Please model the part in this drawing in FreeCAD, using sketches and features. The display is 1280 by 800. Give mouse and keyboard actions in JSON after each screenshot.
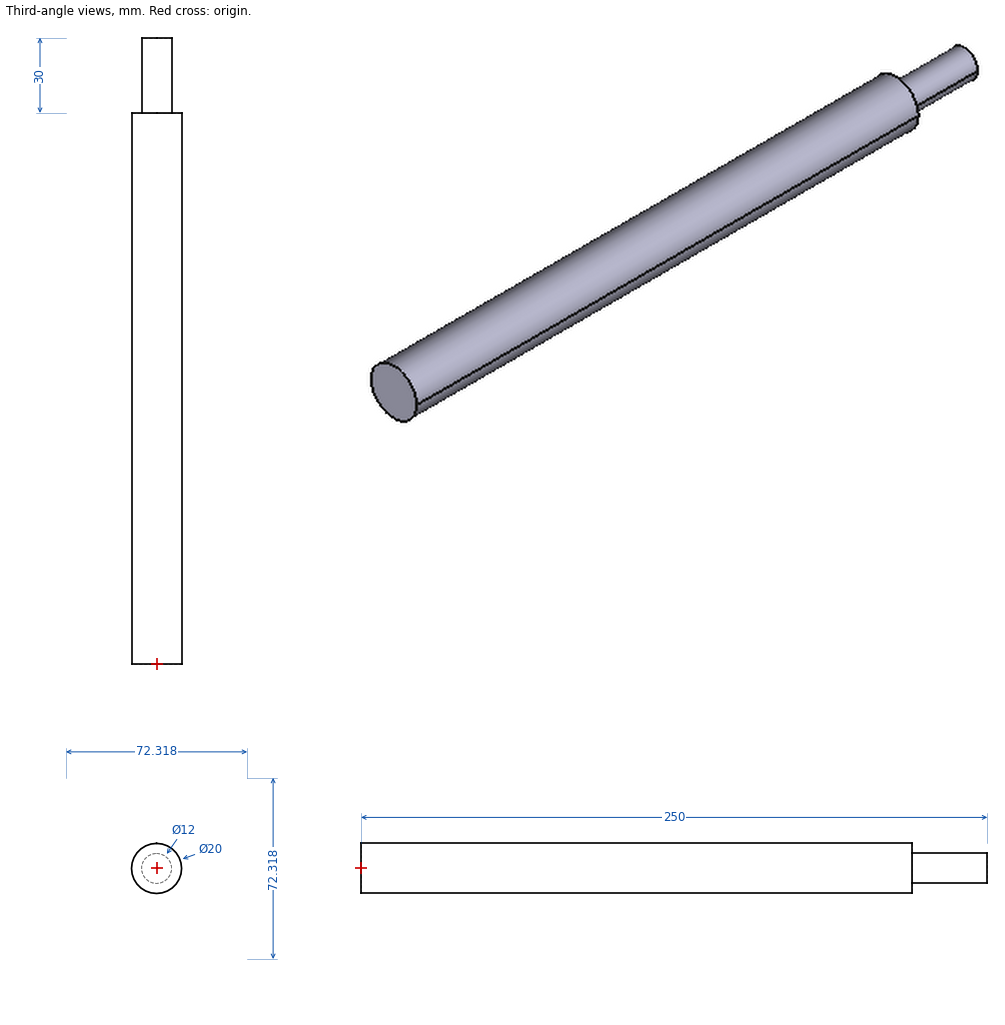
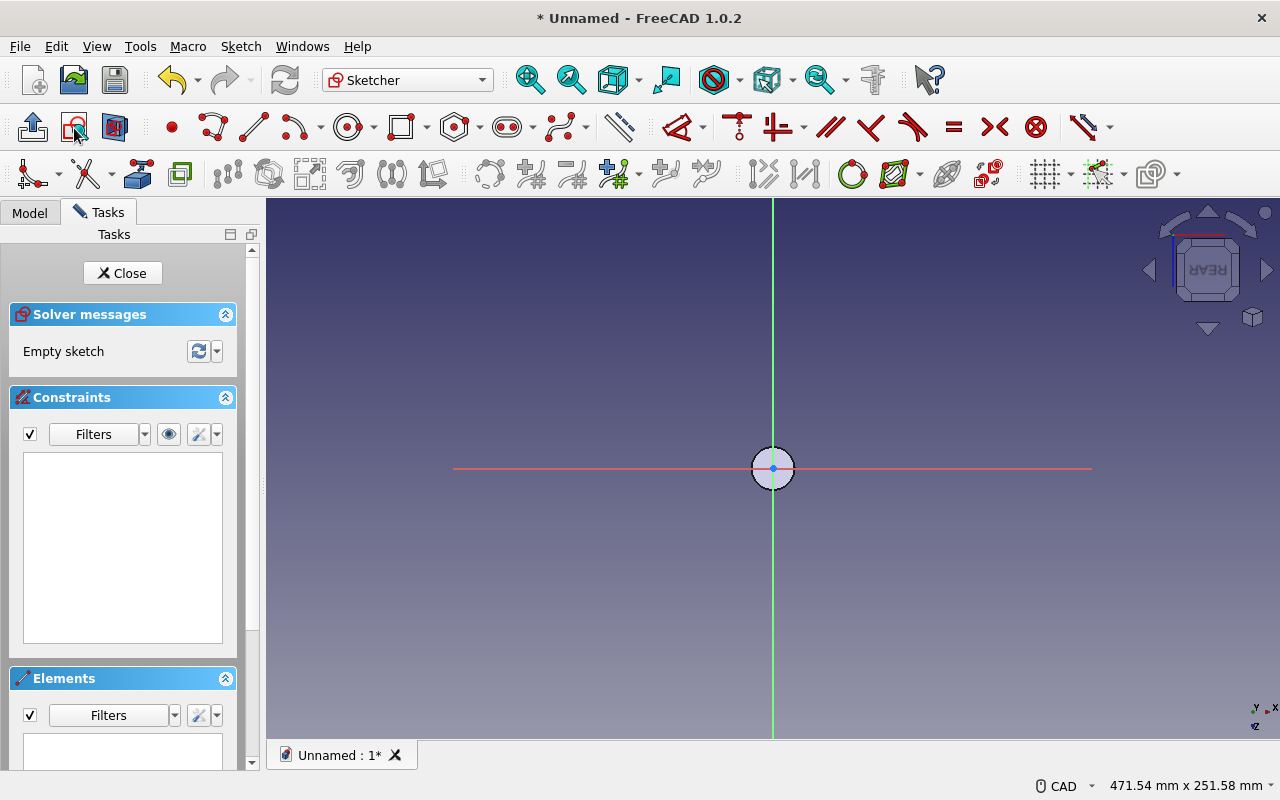
{"action": "scroll", "coordinate": [829, 468], "scroll_direction": "up", "scroll_amount": 4}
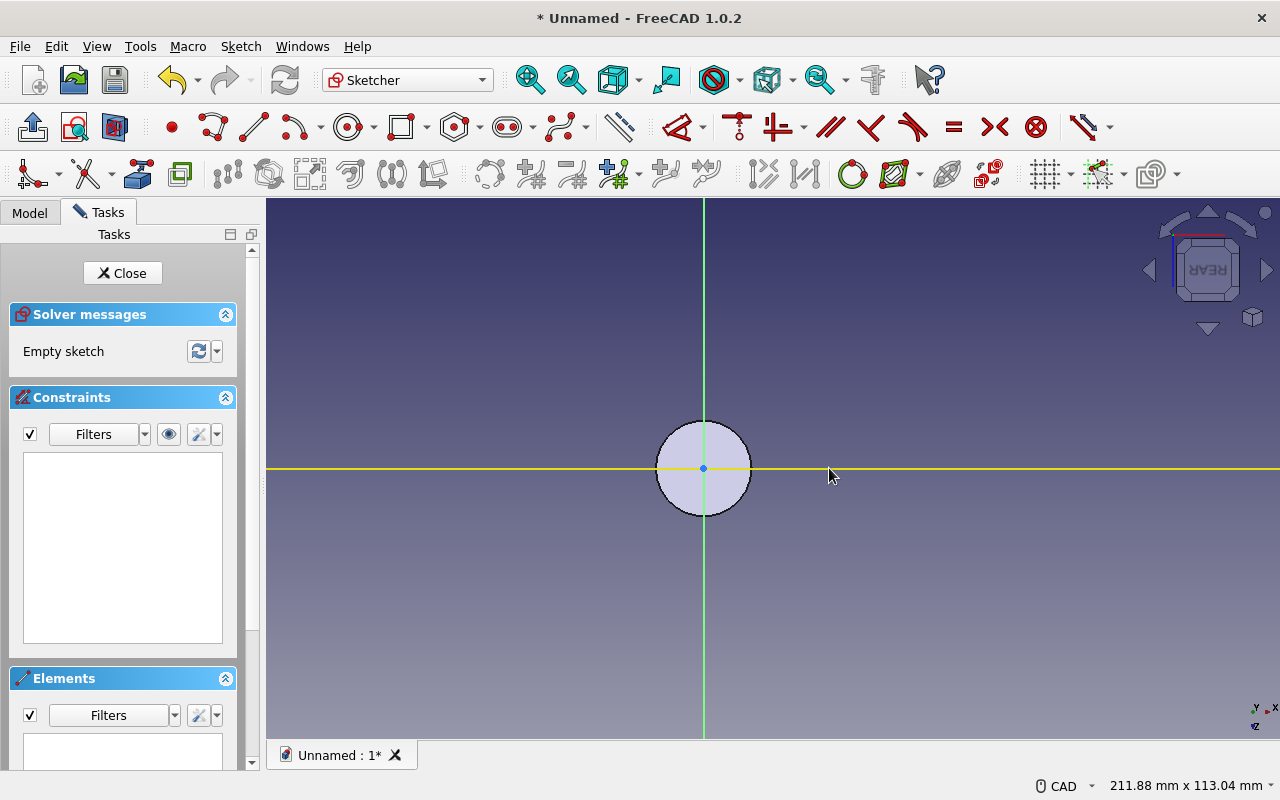
{"action": "key", "text": "g v"}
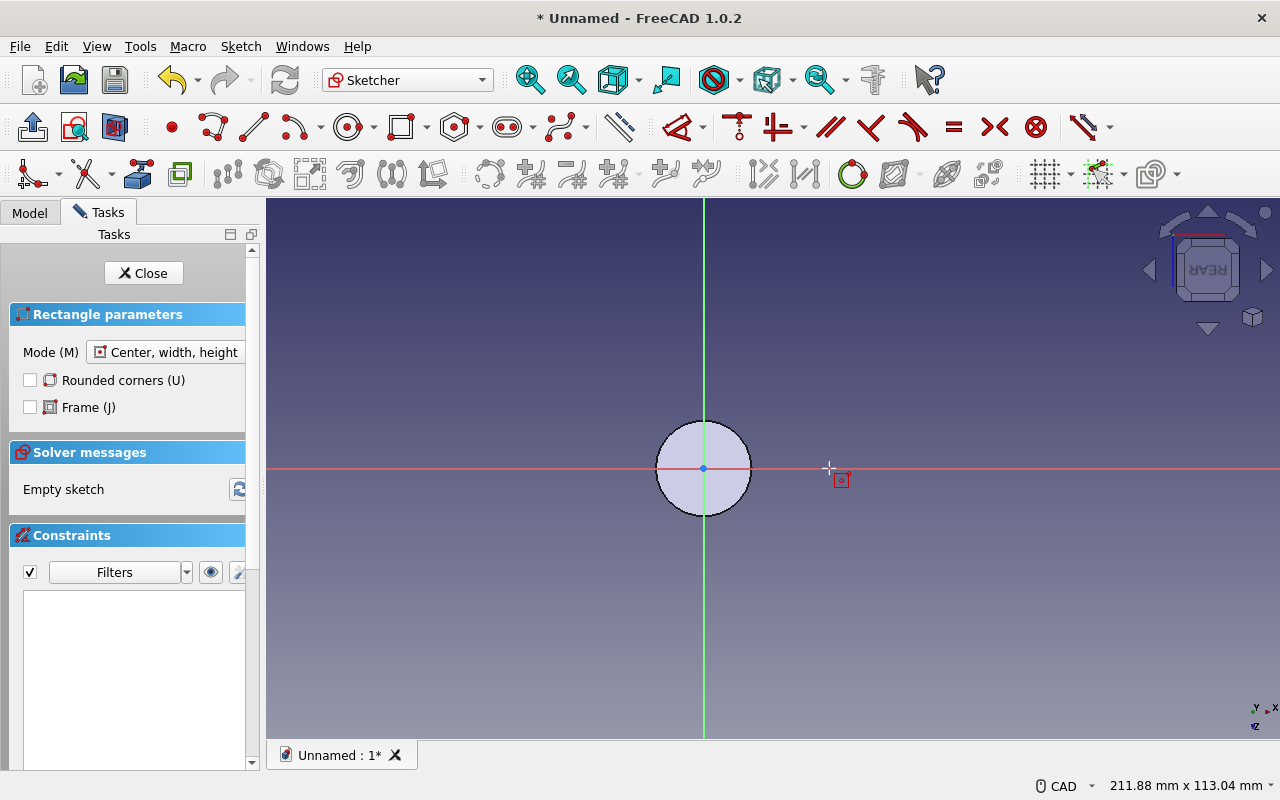
{"action": "left_click", "coordinate": [704, 468]}
{"action": "left_click", "coordinate": [877, 295]}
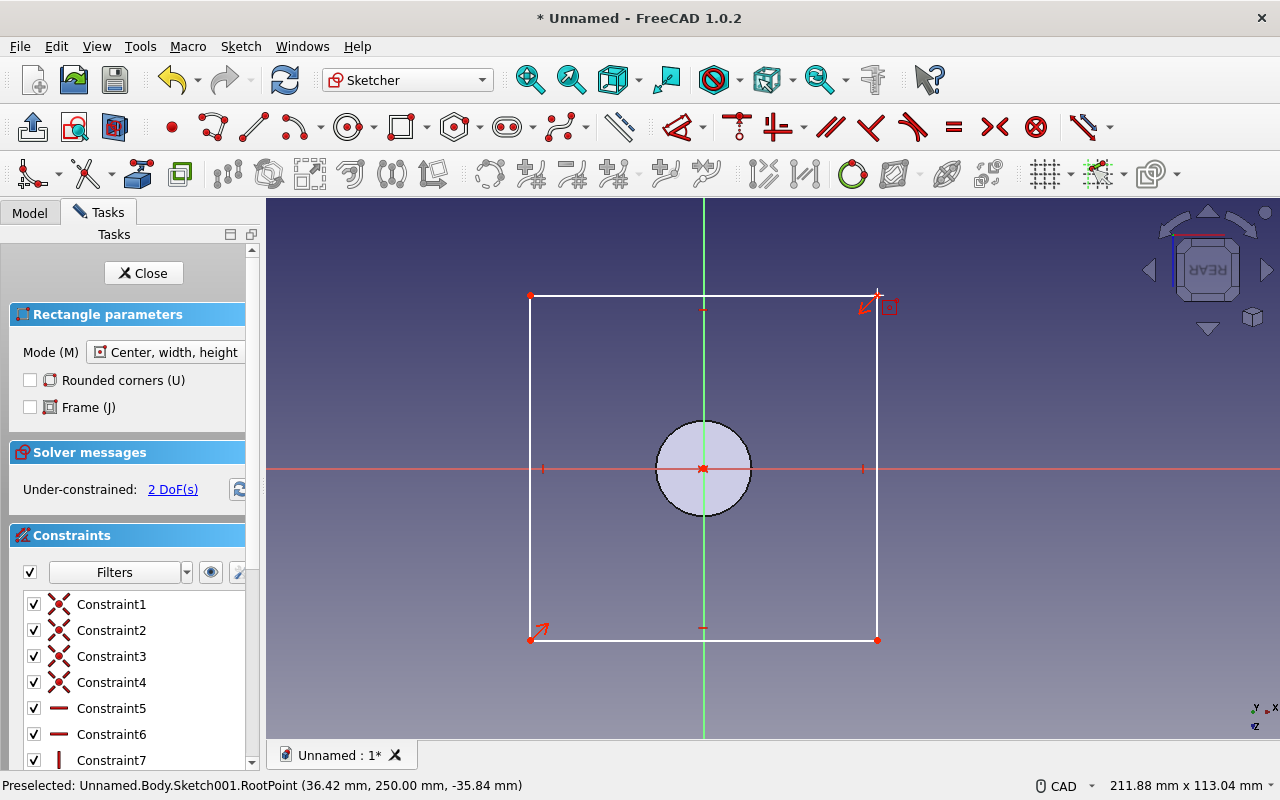
{"action": "left_click", "coordinate": [348, 128]}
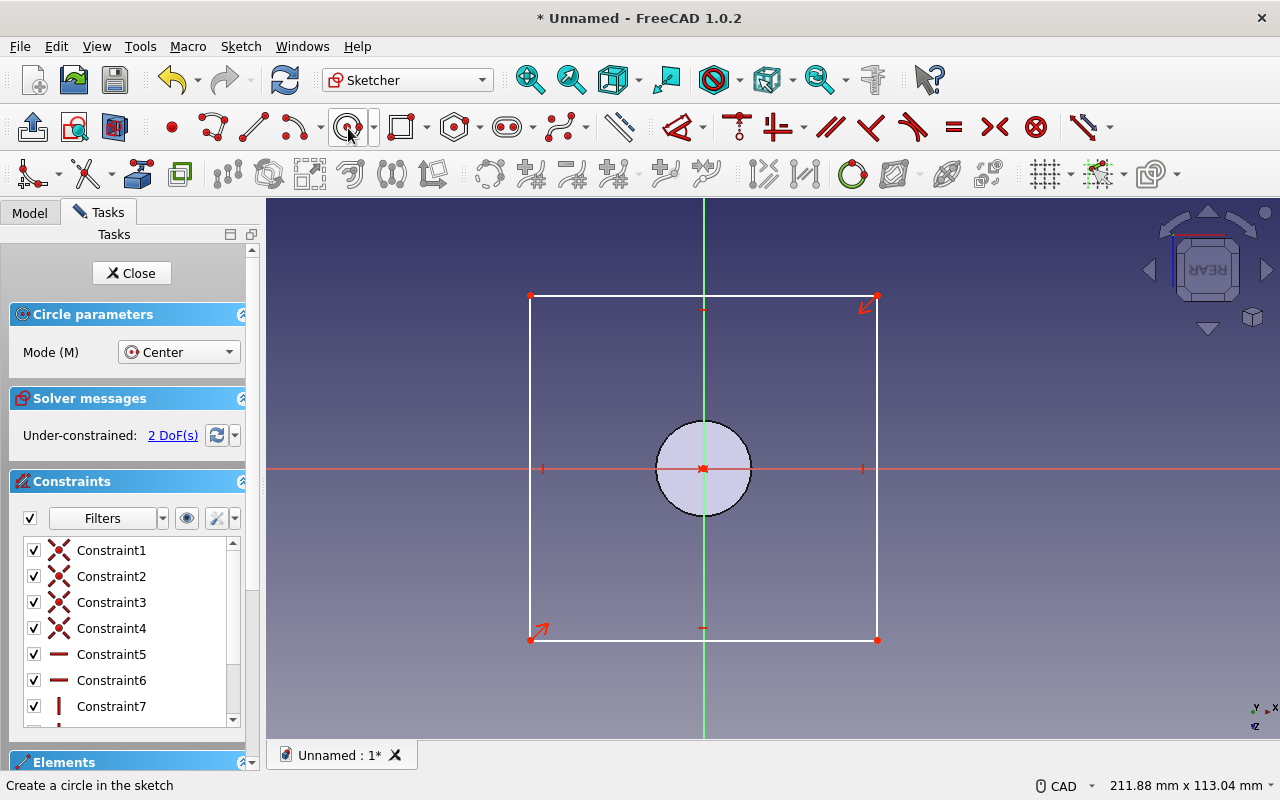
{"action": "left_click", "coordinate": [704, 468]}
{"action": "left_click", "coordinate": [724, 448]}
{"action": "key", "text": "Escape"}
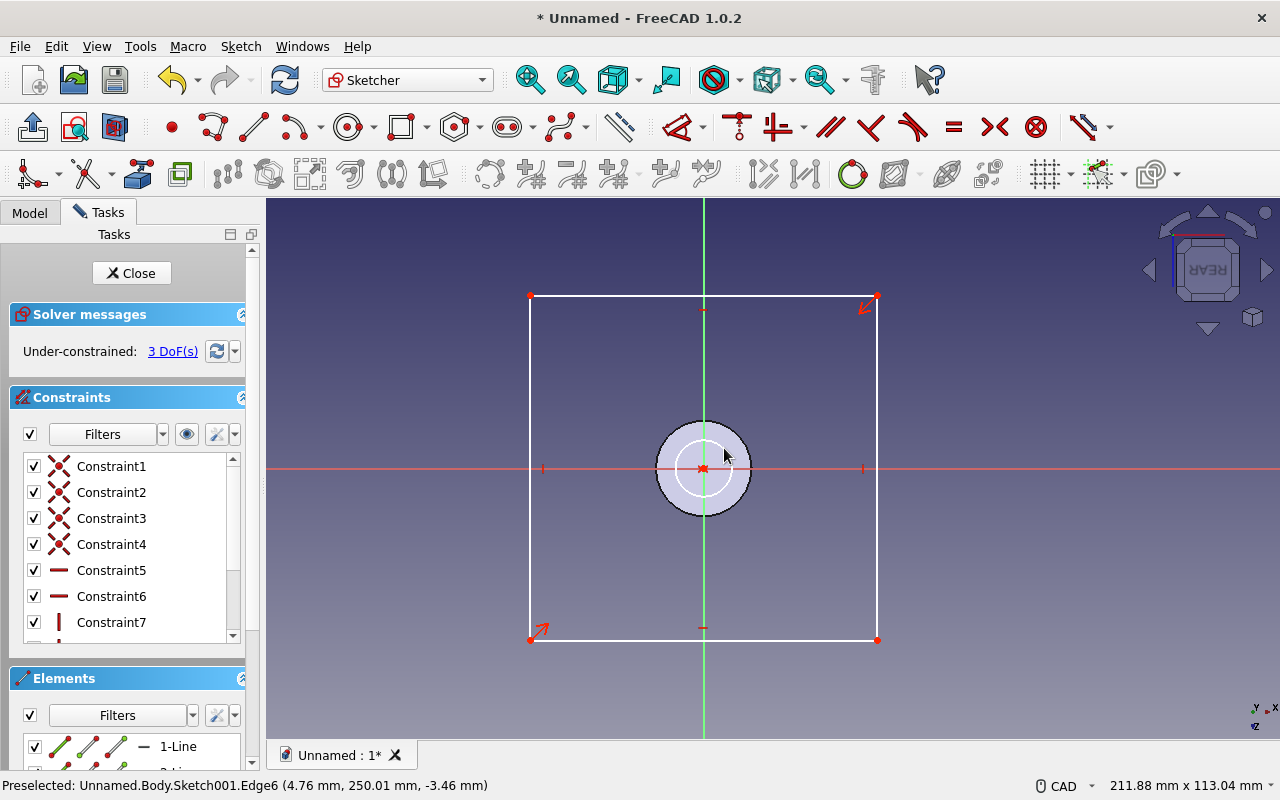
{"action": "left_click", "coordinate": [676, 128]}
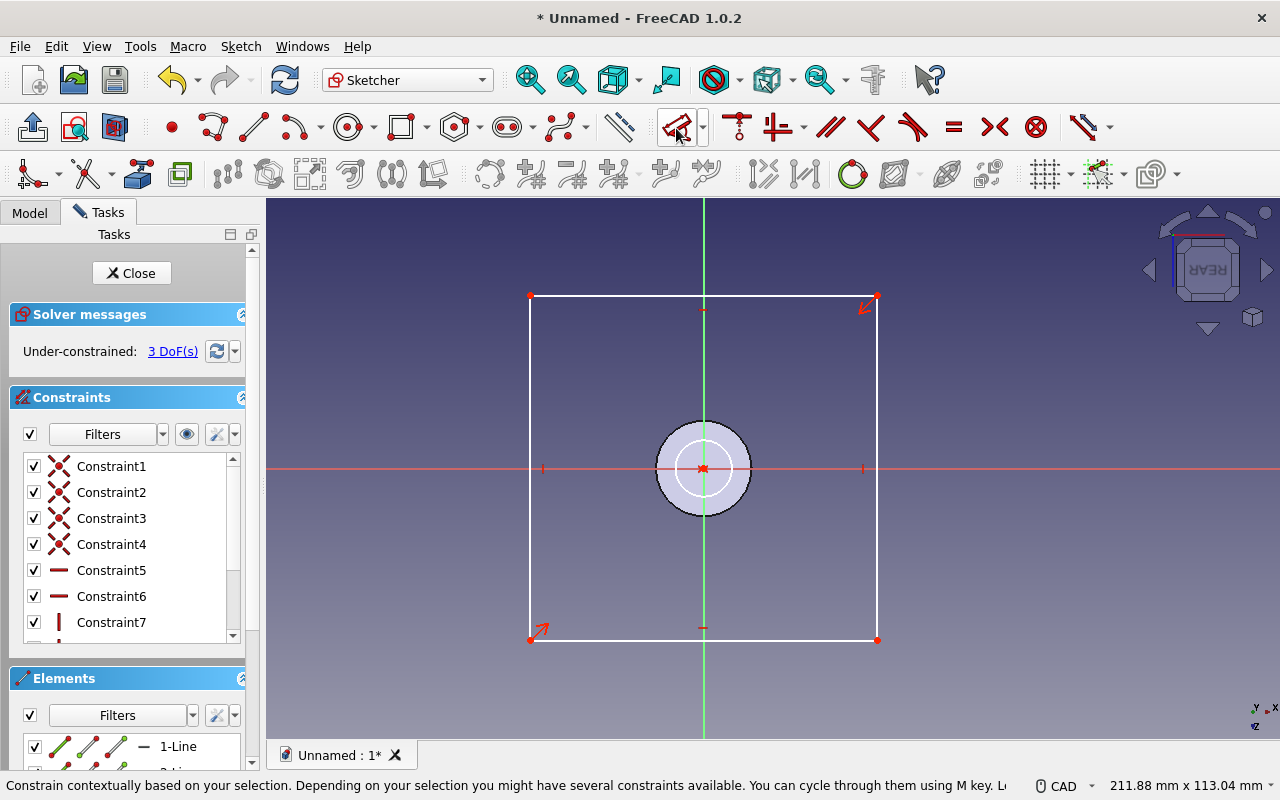
{"action": "left_click", "coordinate": [724, 449]}
{"action": "left_click", "coordinate": [747, 427]}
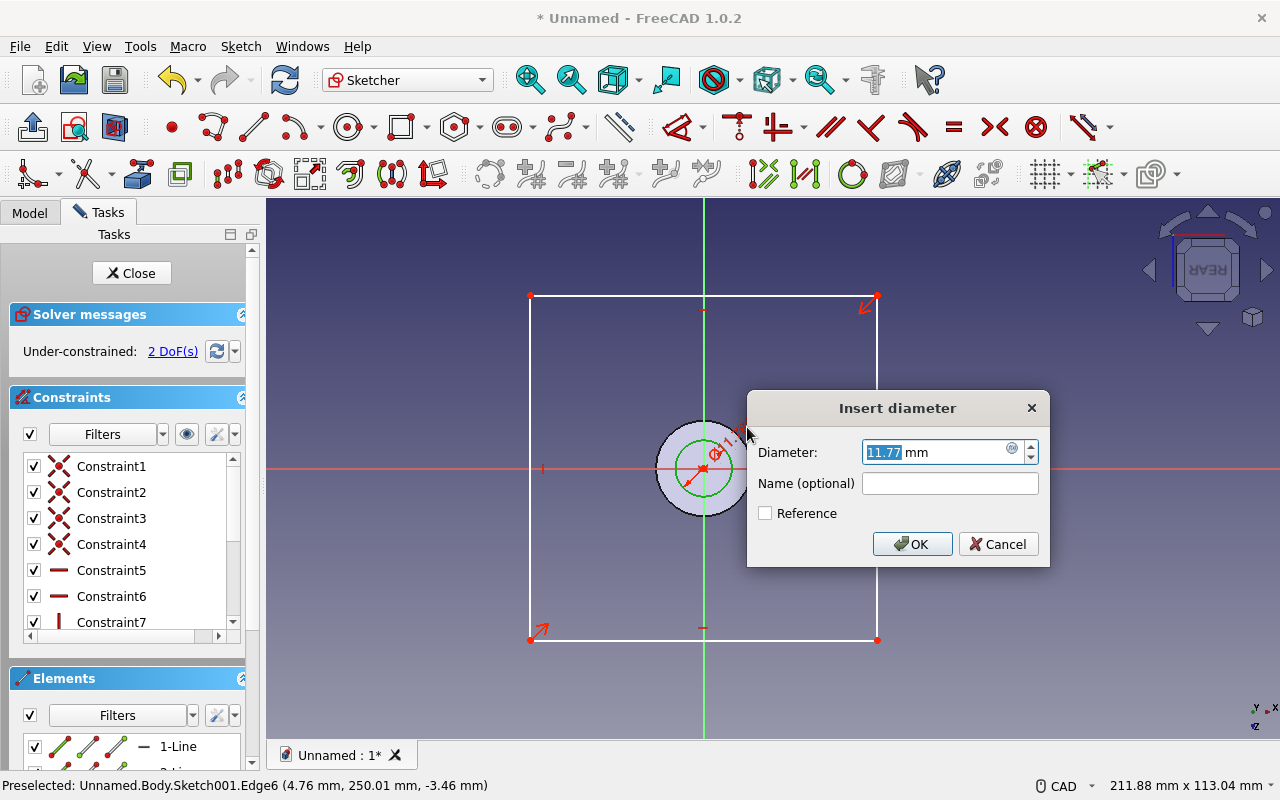
{"action": "type", "text": "12"}
{"action": "key", "text": "Return"}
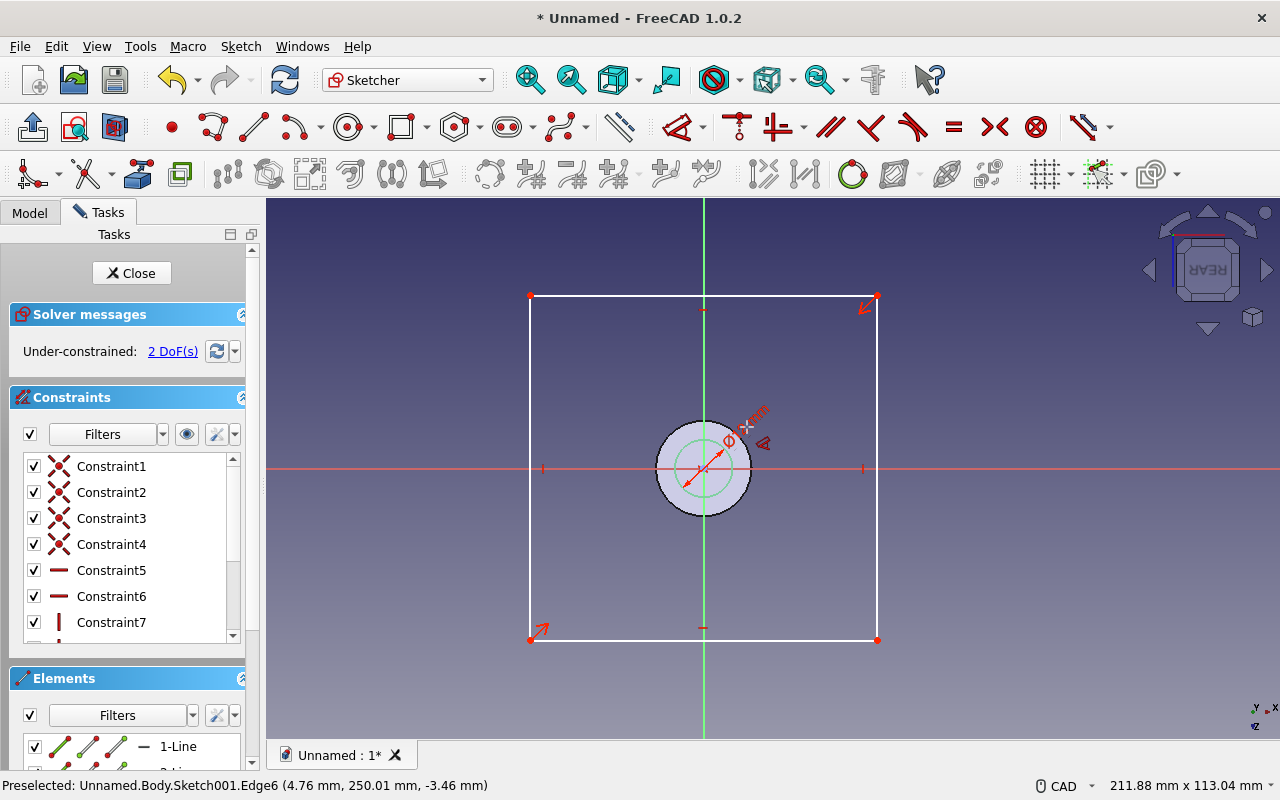
{"action": "left_click", "coordinate": [634, 641]}
{"action": "left_click", "coordinate": [624, 675]}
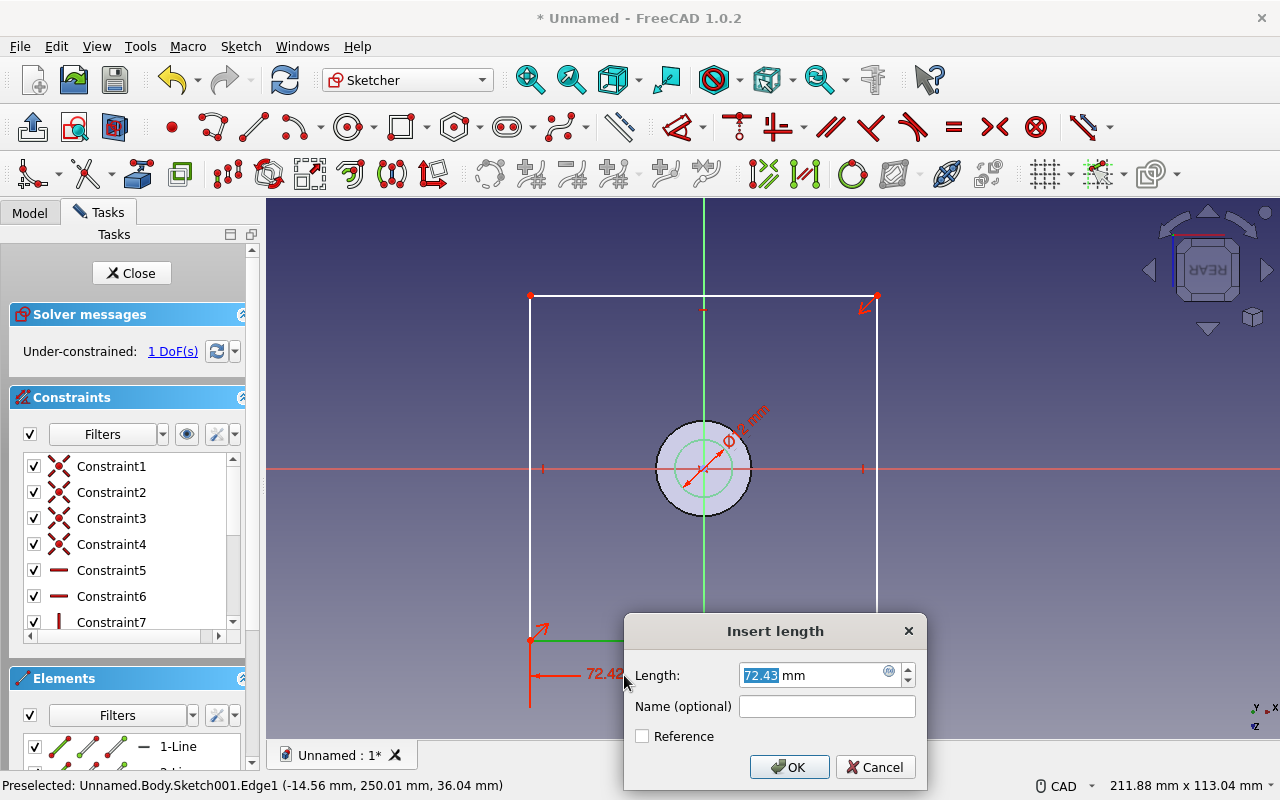
{"action": "type", "text": "72.318"}
{"action": "key", "text": "Return"}